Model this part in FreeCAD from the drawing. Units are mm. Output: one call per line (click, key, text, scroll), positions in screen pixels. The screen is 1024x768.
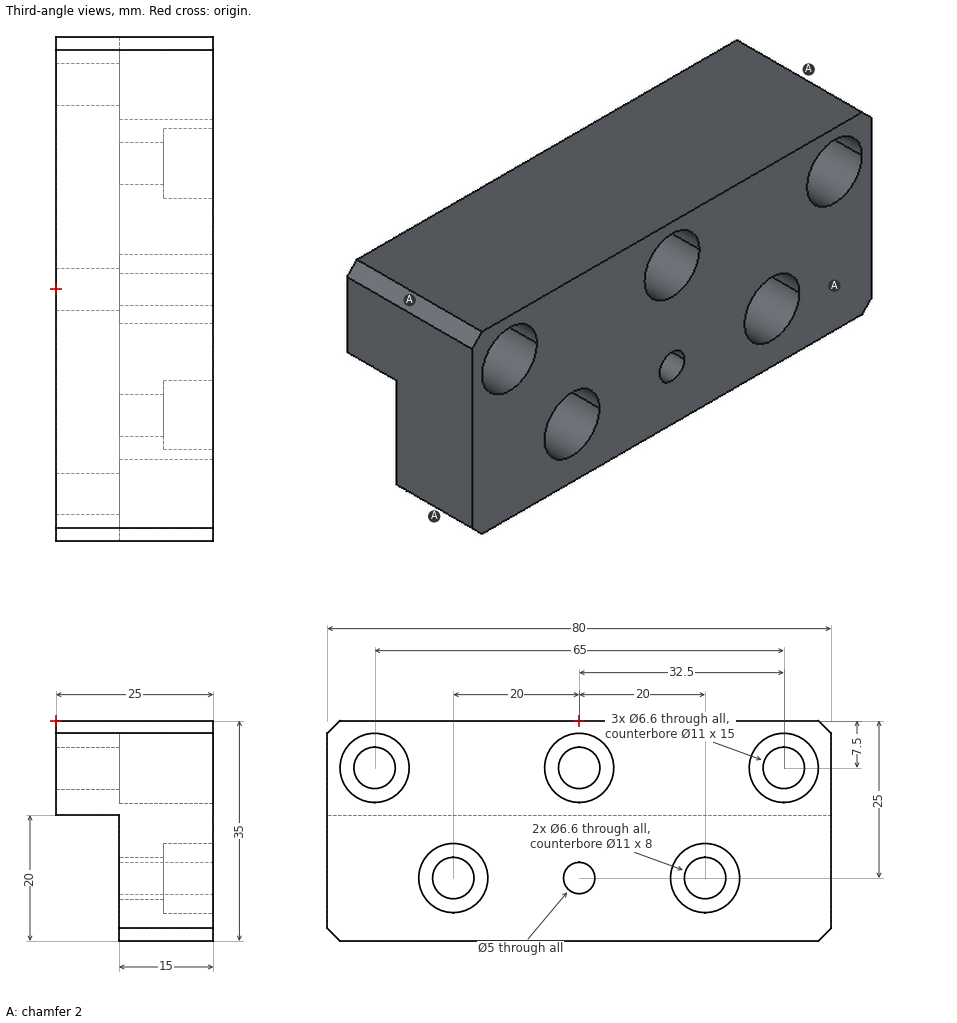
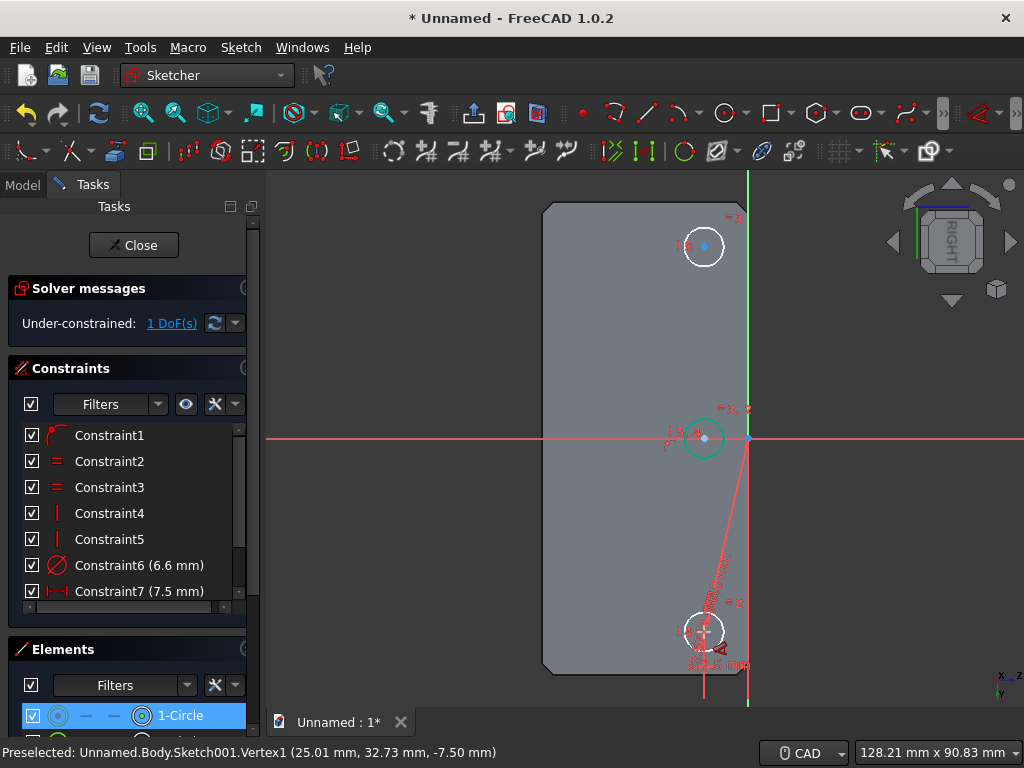
click(704, 247)
click(670, 351)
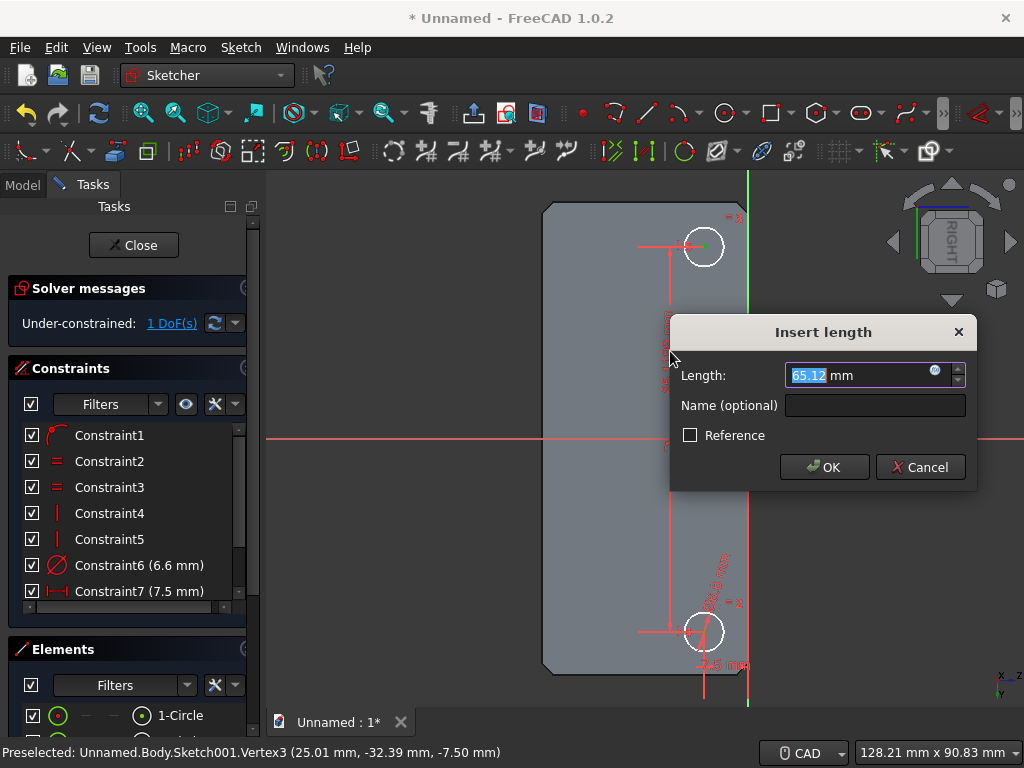
text(65)
key(Return)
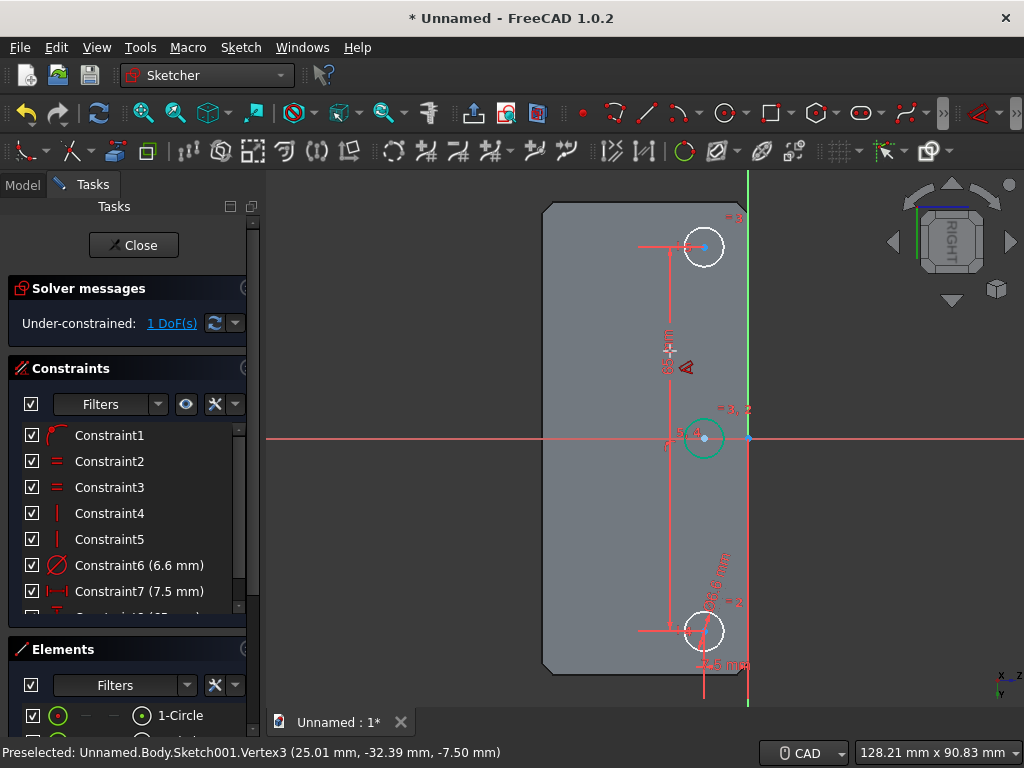
click(704, 631)
click(782, 535)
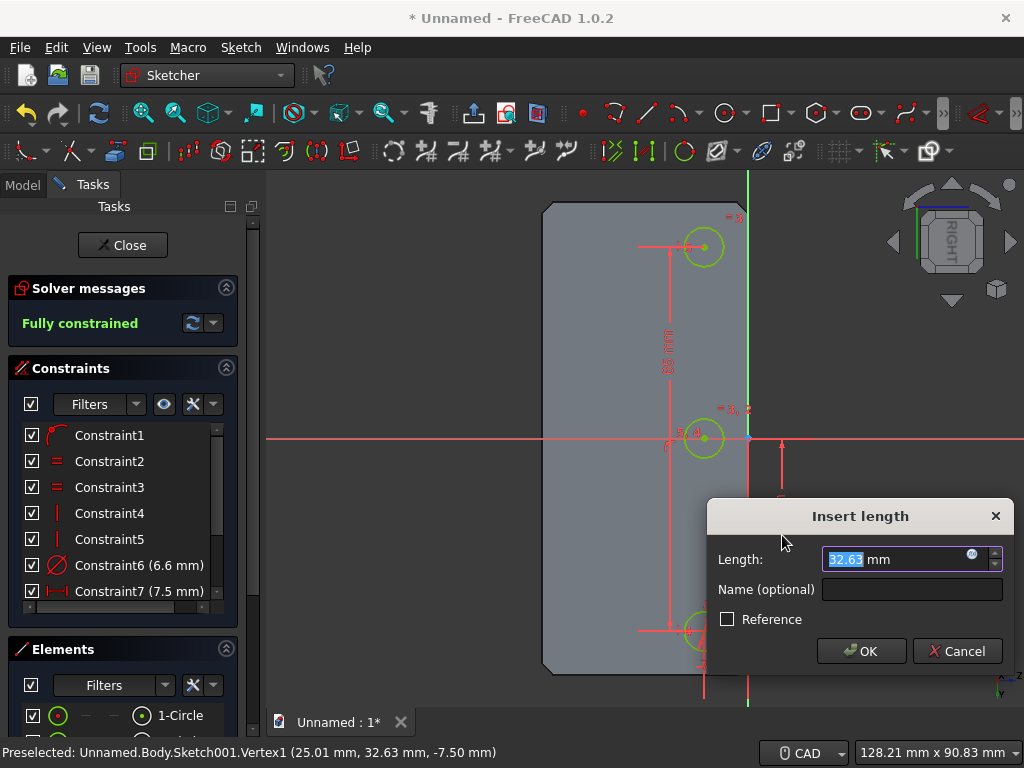
text(32.5)
key(Return)
key(Escape)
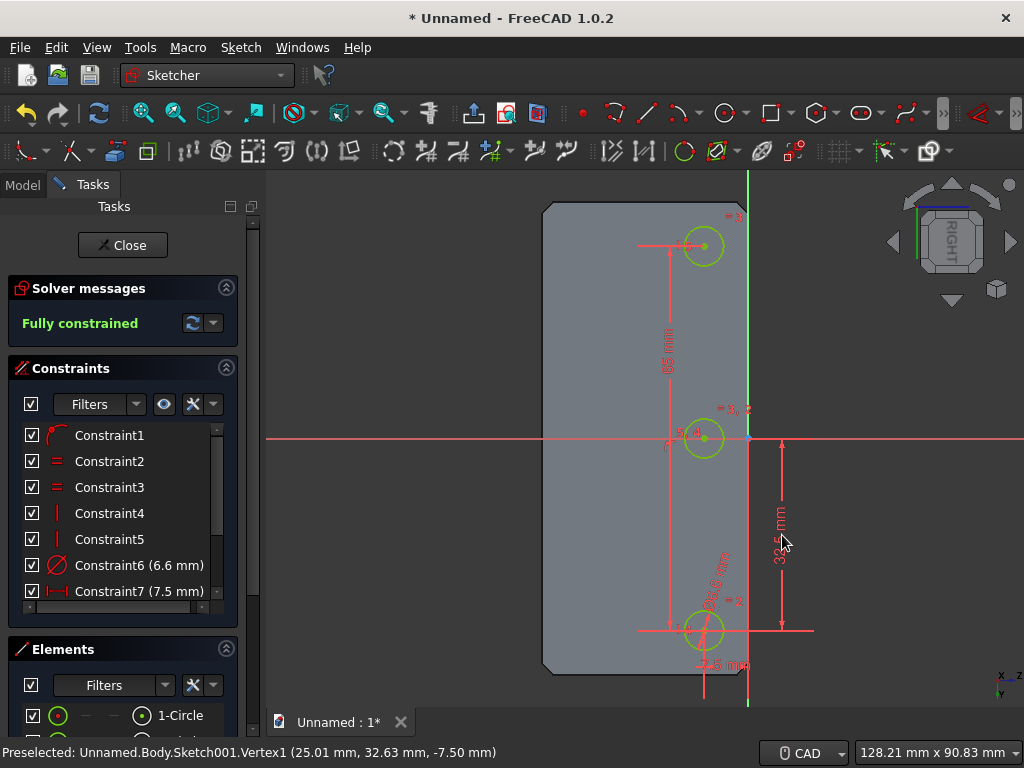
click(123, 245)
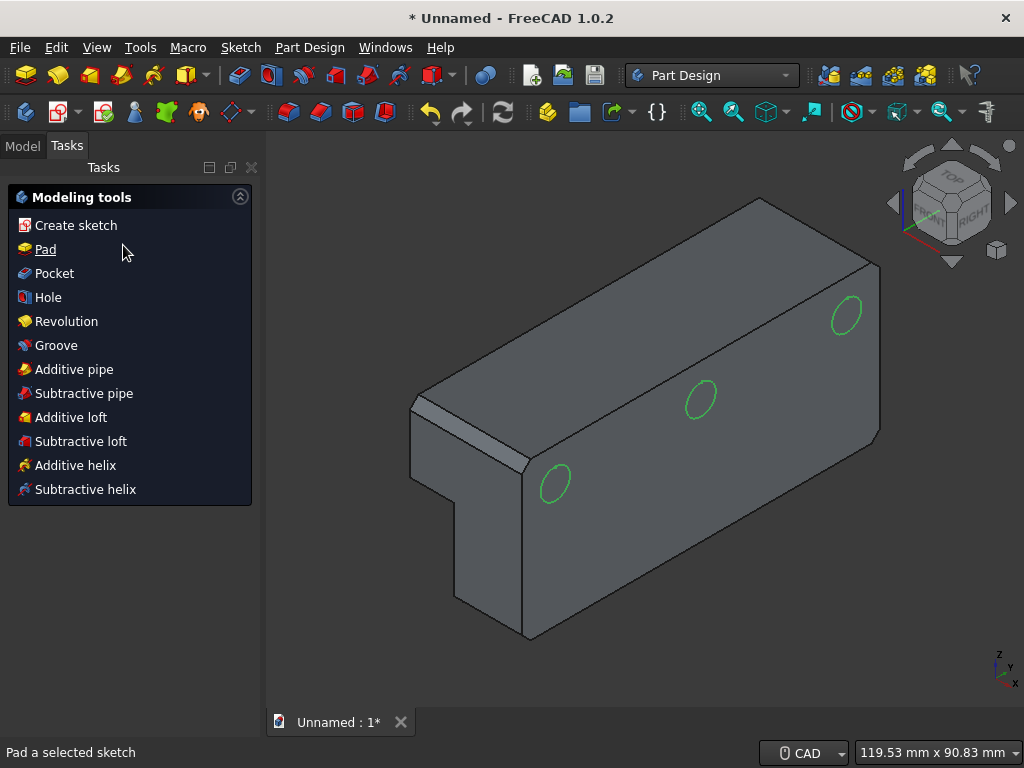
click(272, 76)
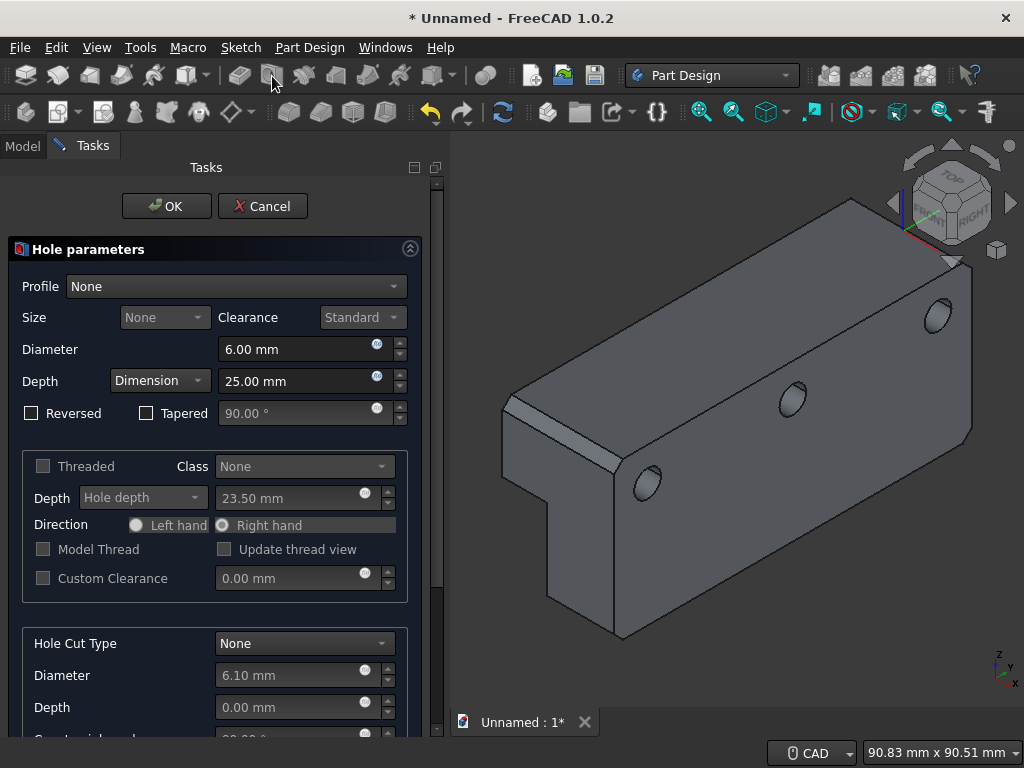
triple_click(305, 349)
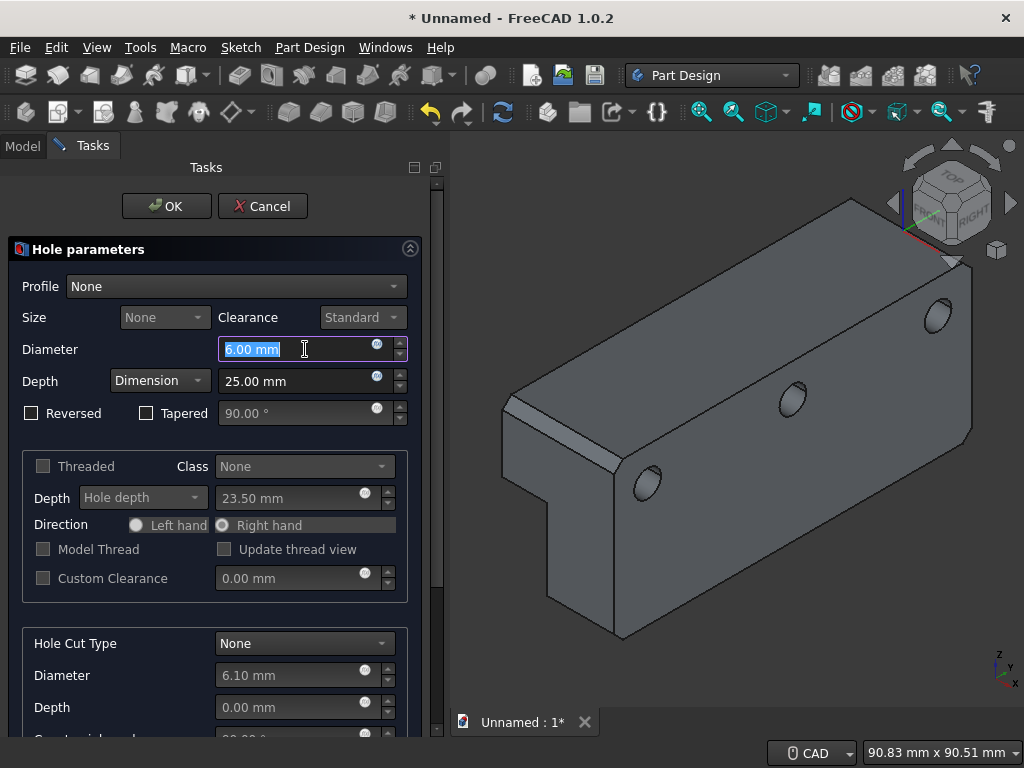
text(6.6)
key(Tab)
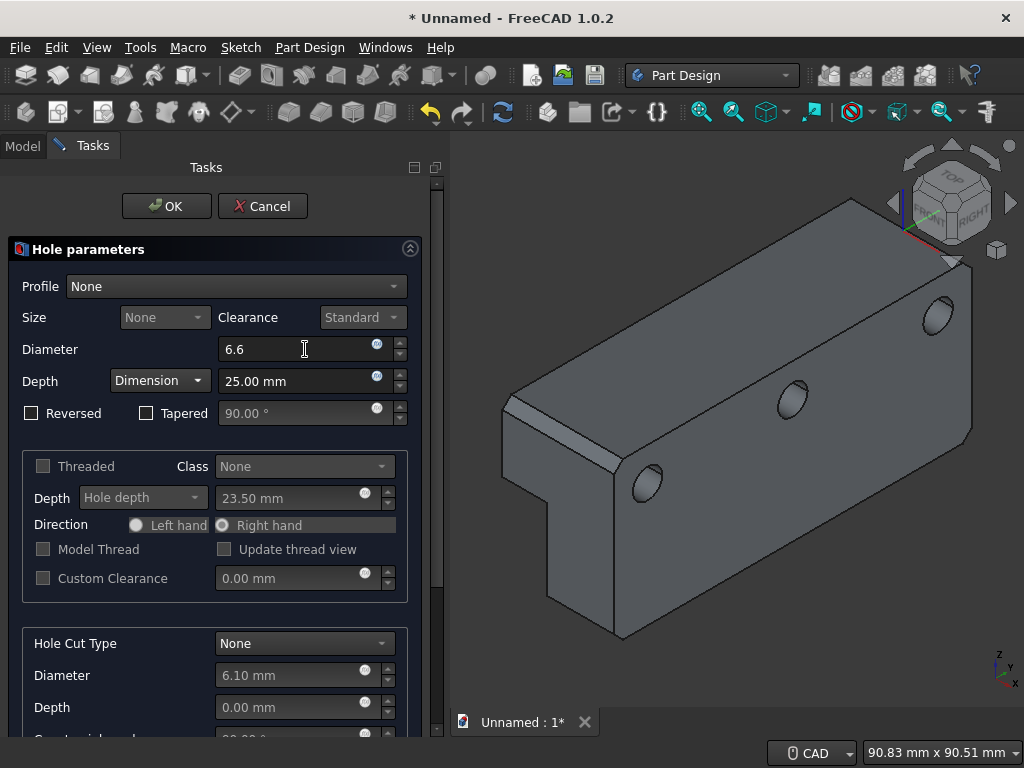
click(161, 380)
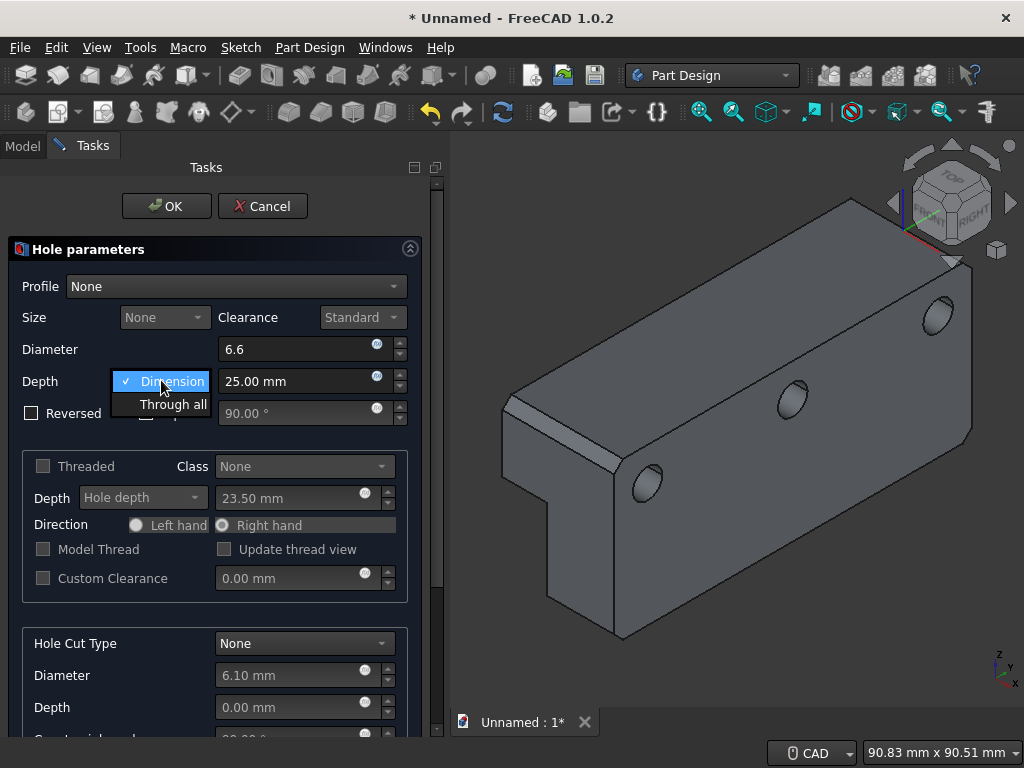
click(160, 404)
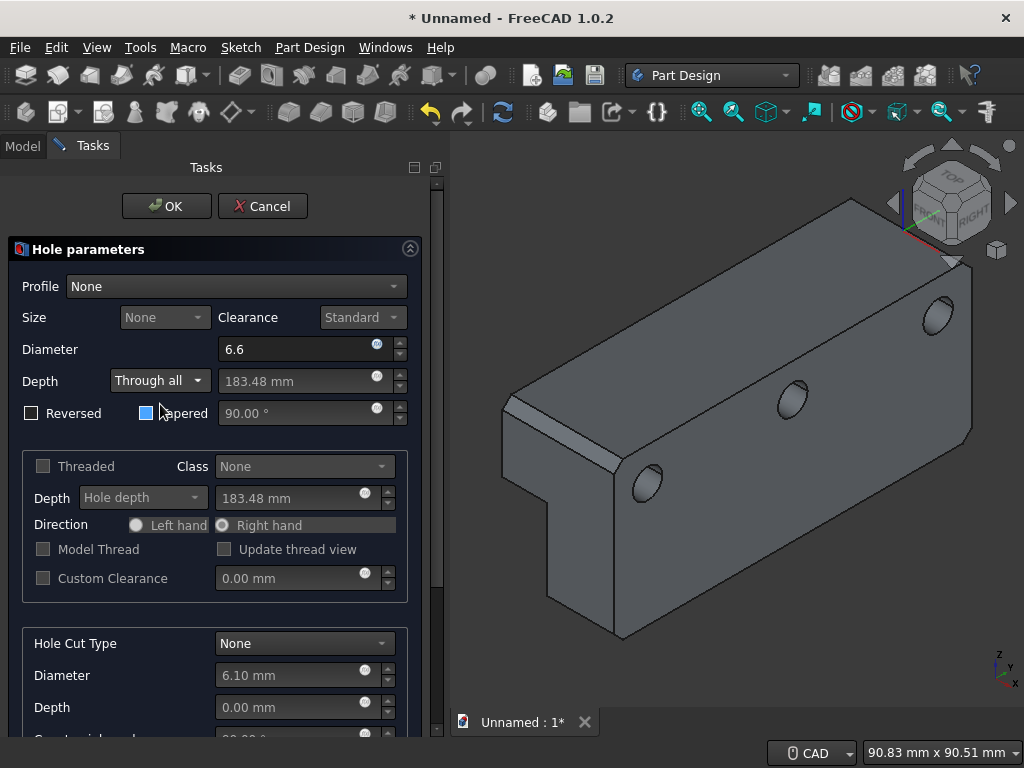
click(306, 644)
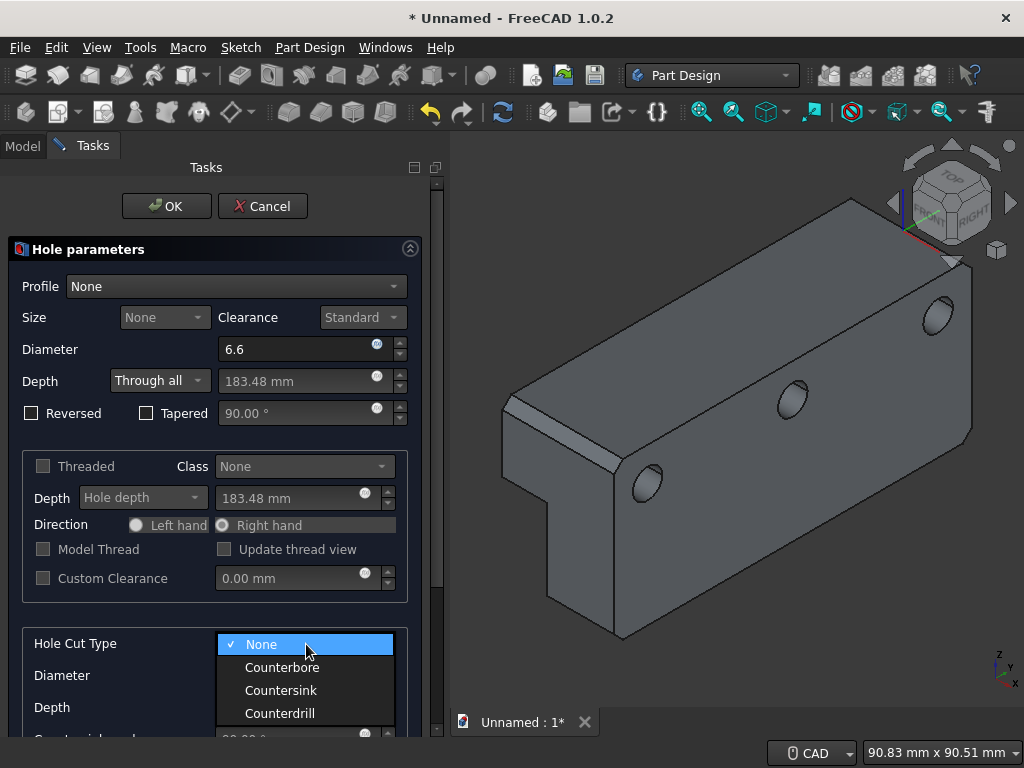
click(304, 668)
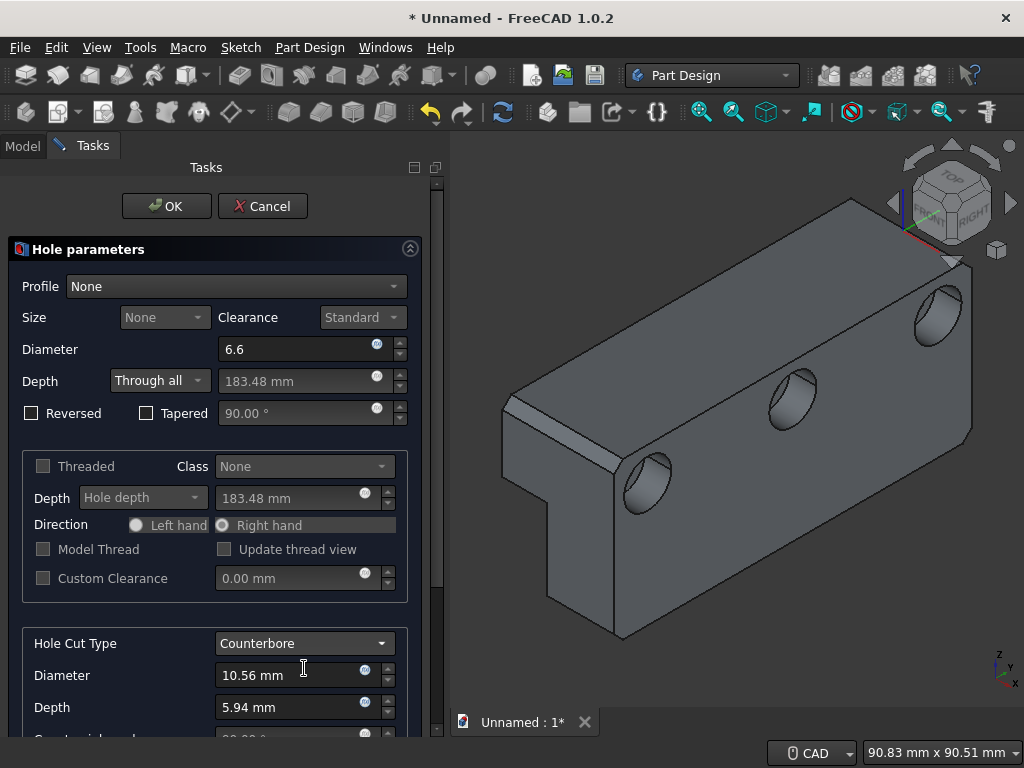
triple_click(298, 675)